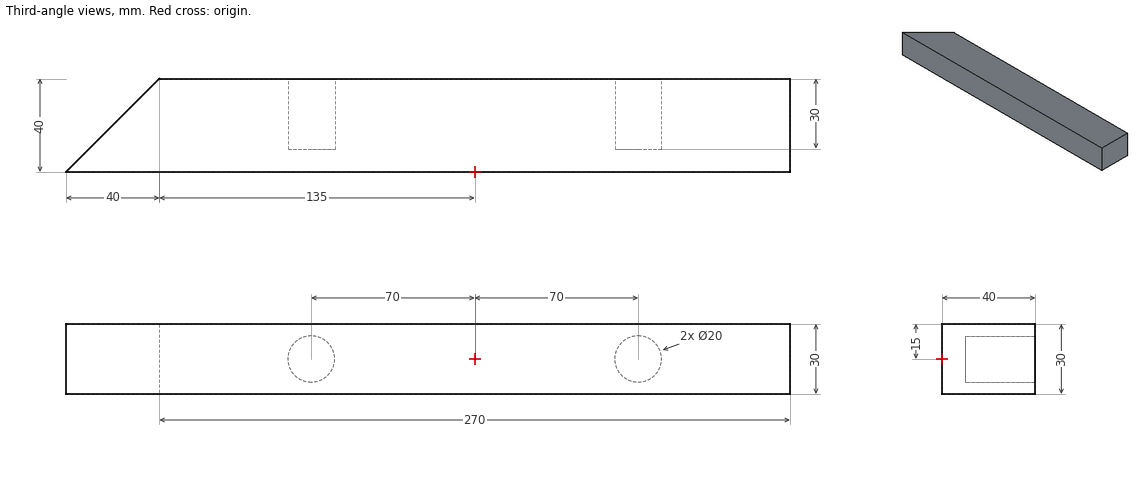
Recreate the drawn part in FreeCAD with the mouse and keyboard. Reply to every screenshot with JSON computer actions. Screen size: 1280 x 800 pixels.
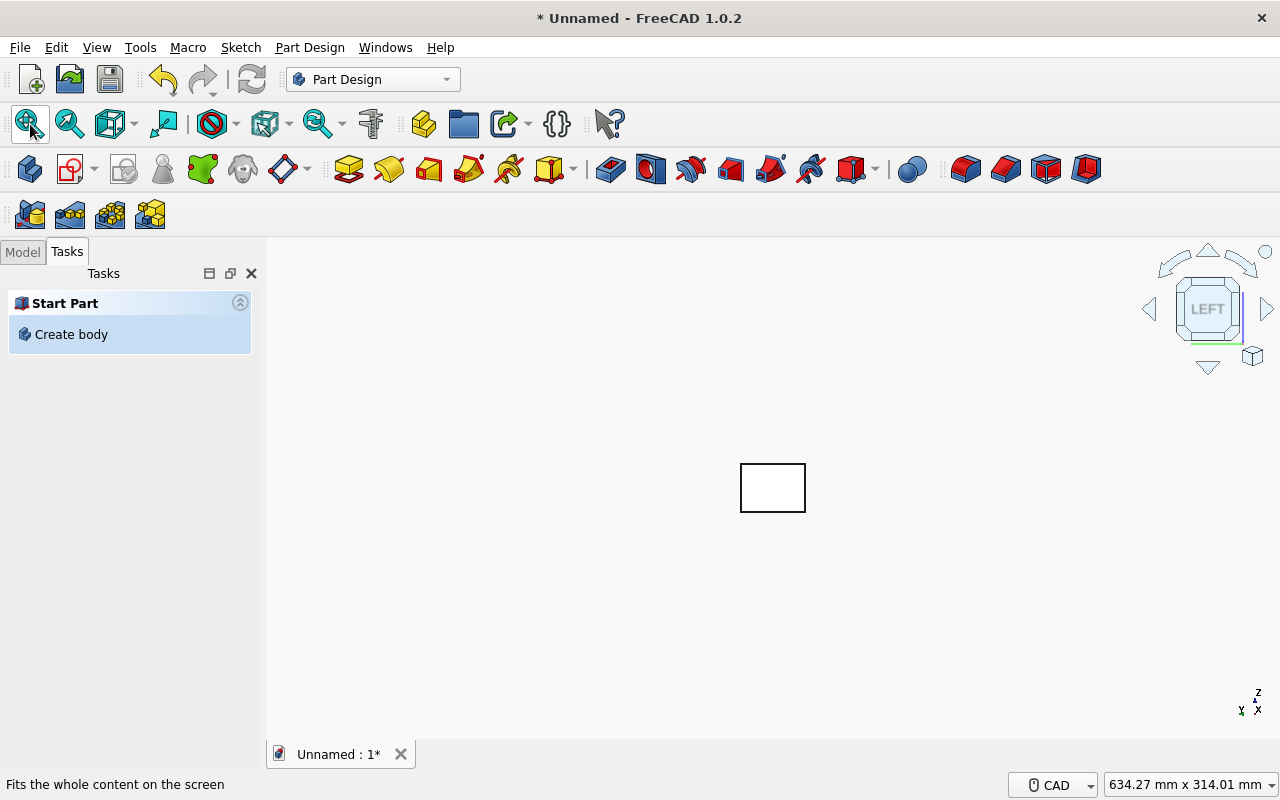
{"action": "key", "text": "0"}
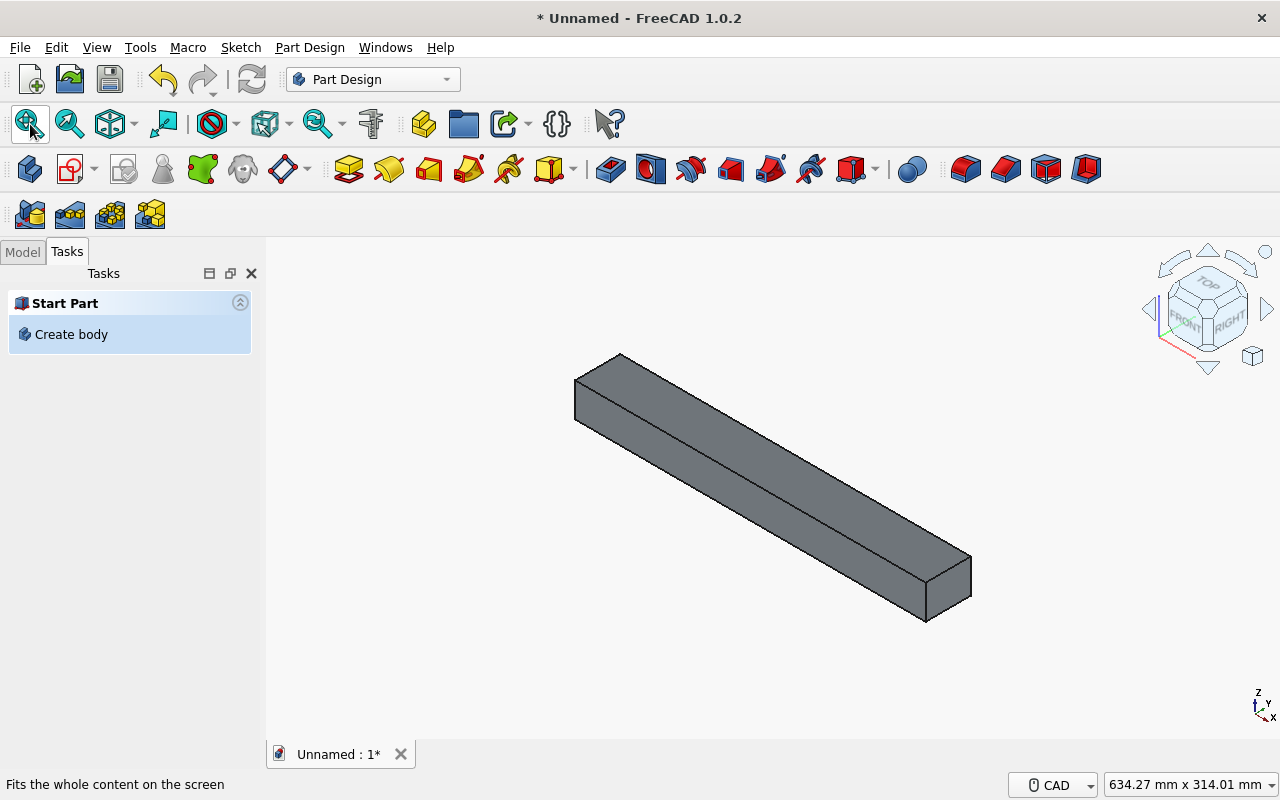
{"action": "left_click", "coordinate": [923, 554]}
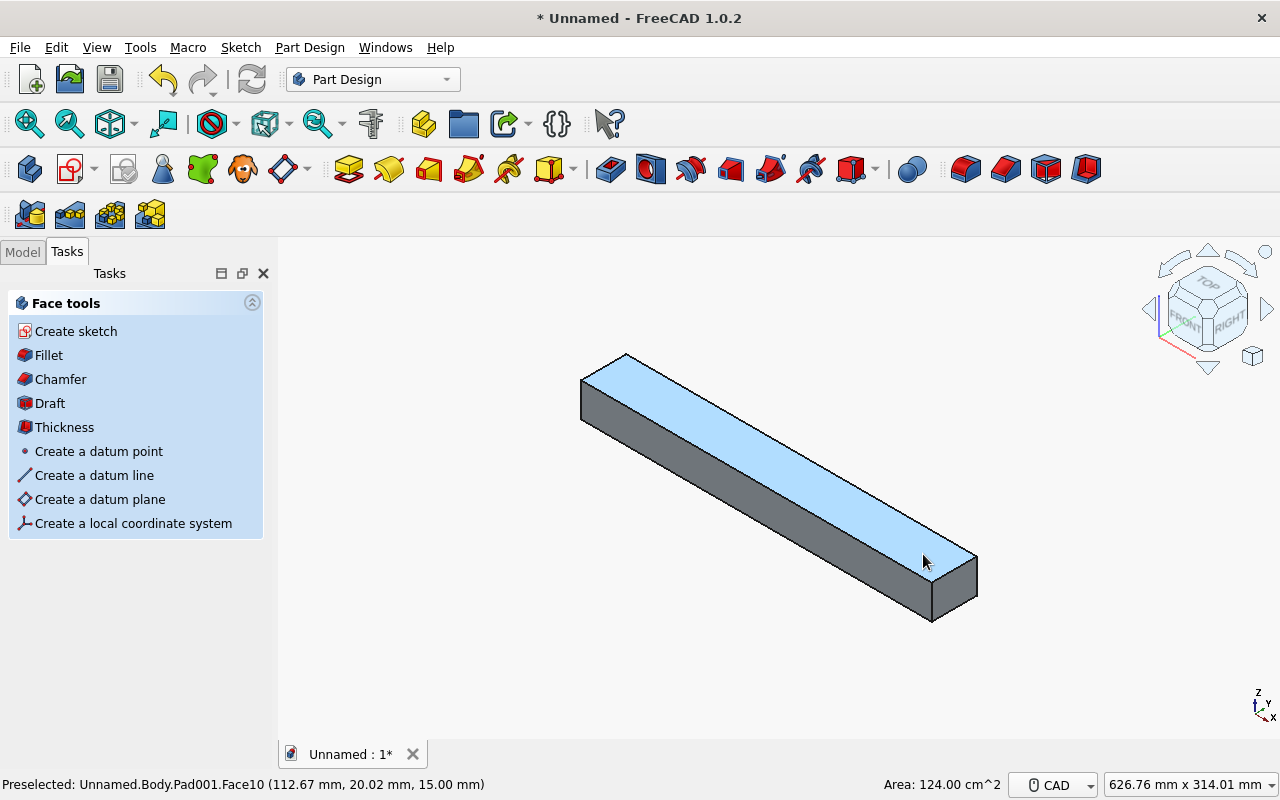
{"action": "left_click", "coordinate": [70, 170]}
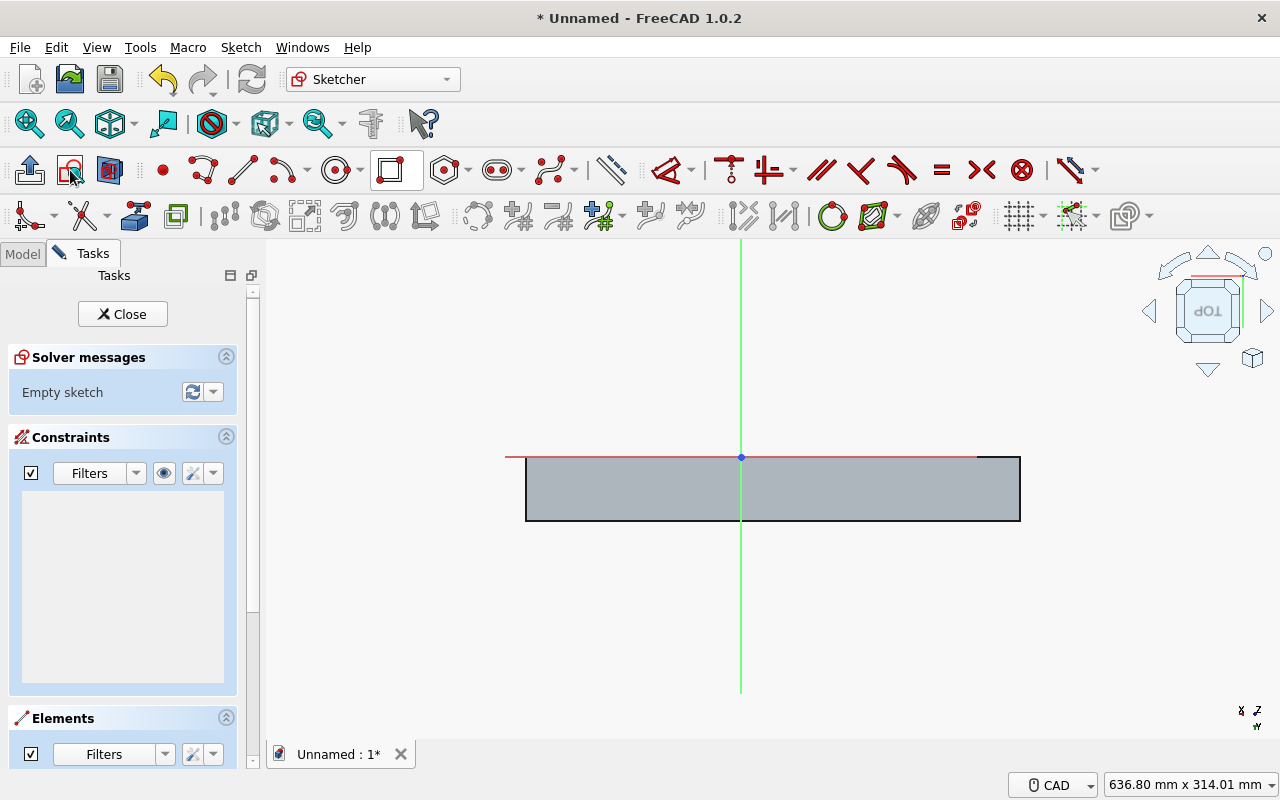
{"action": "scroll", "coordinate": [1060, 489], "scroll_direction": "up", "scroll_amount": 8}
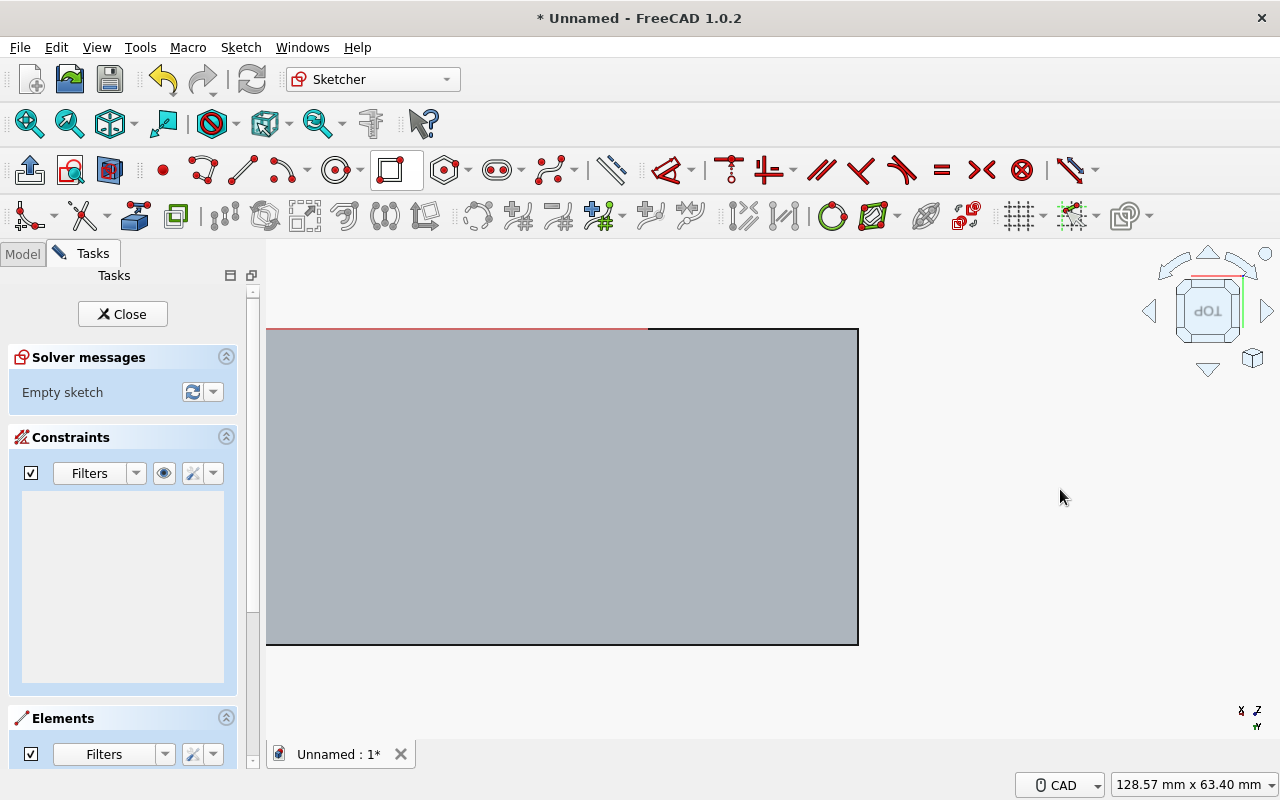
{"action": "left_click", "coordinate": [204, 170]}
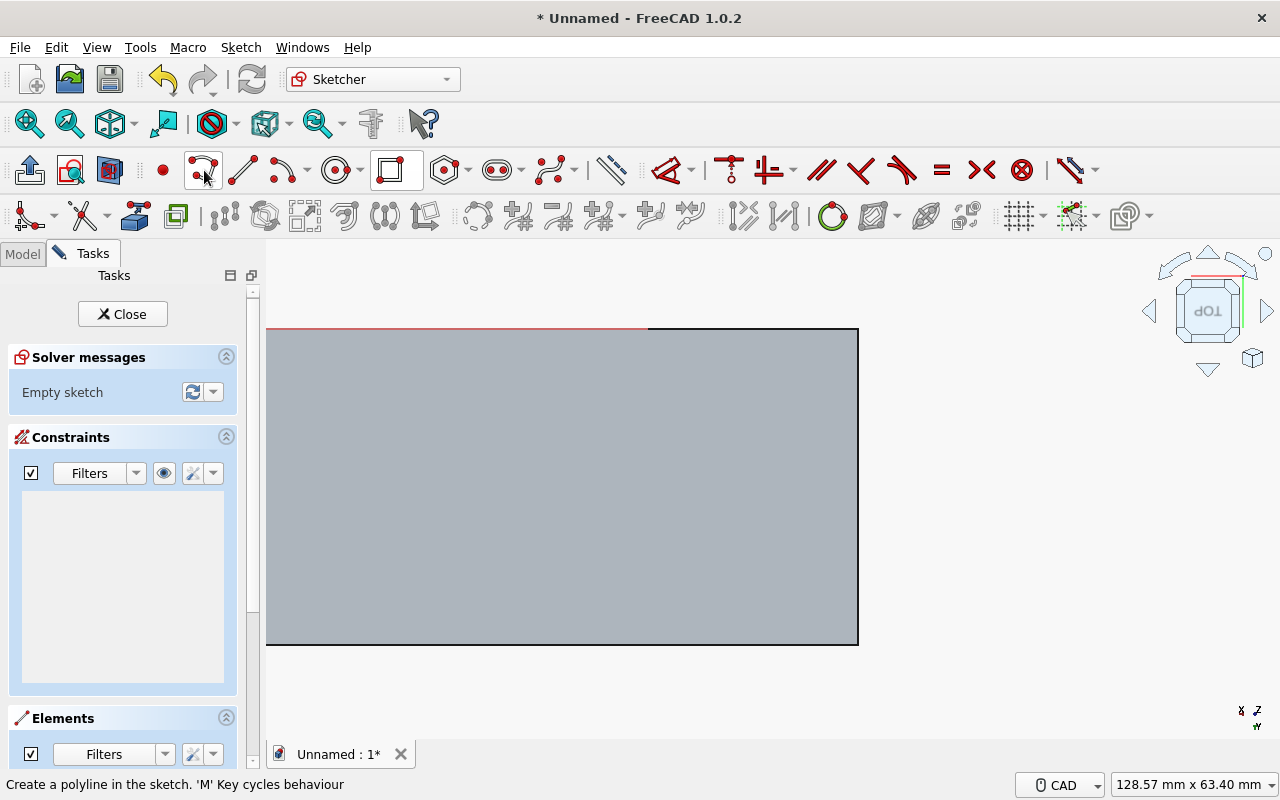
{"action": "left_click", "coordinate": [542, 645]}
{"action": "left_click", "coordinate": [858, 645]}
{"action": "left_click", "coordinate": [858, 329]}
{"action": "left_click", "coordinate": [542, 646]}
{"action": "key", "text": "Escape"}
{"action": "key", "text": "Escape"}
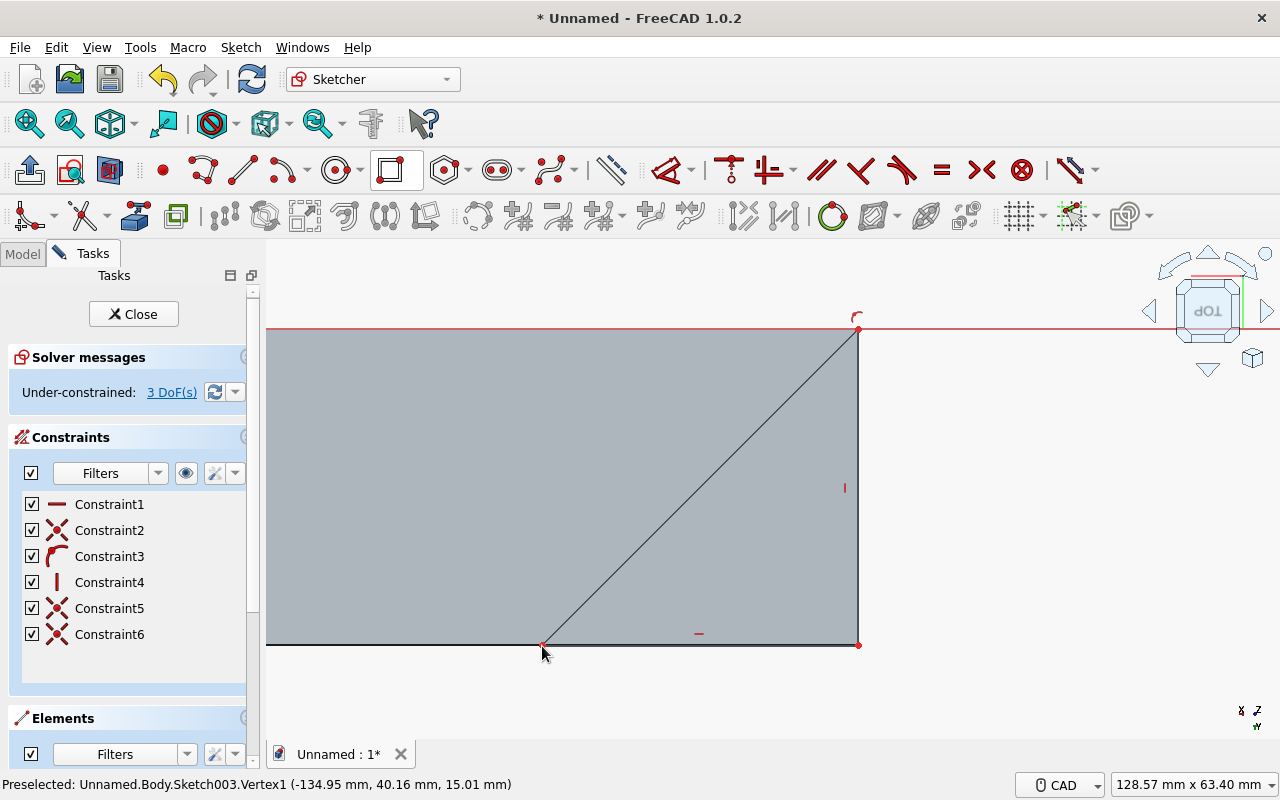
{"action": "left_click", "coordinate": [666, 170]}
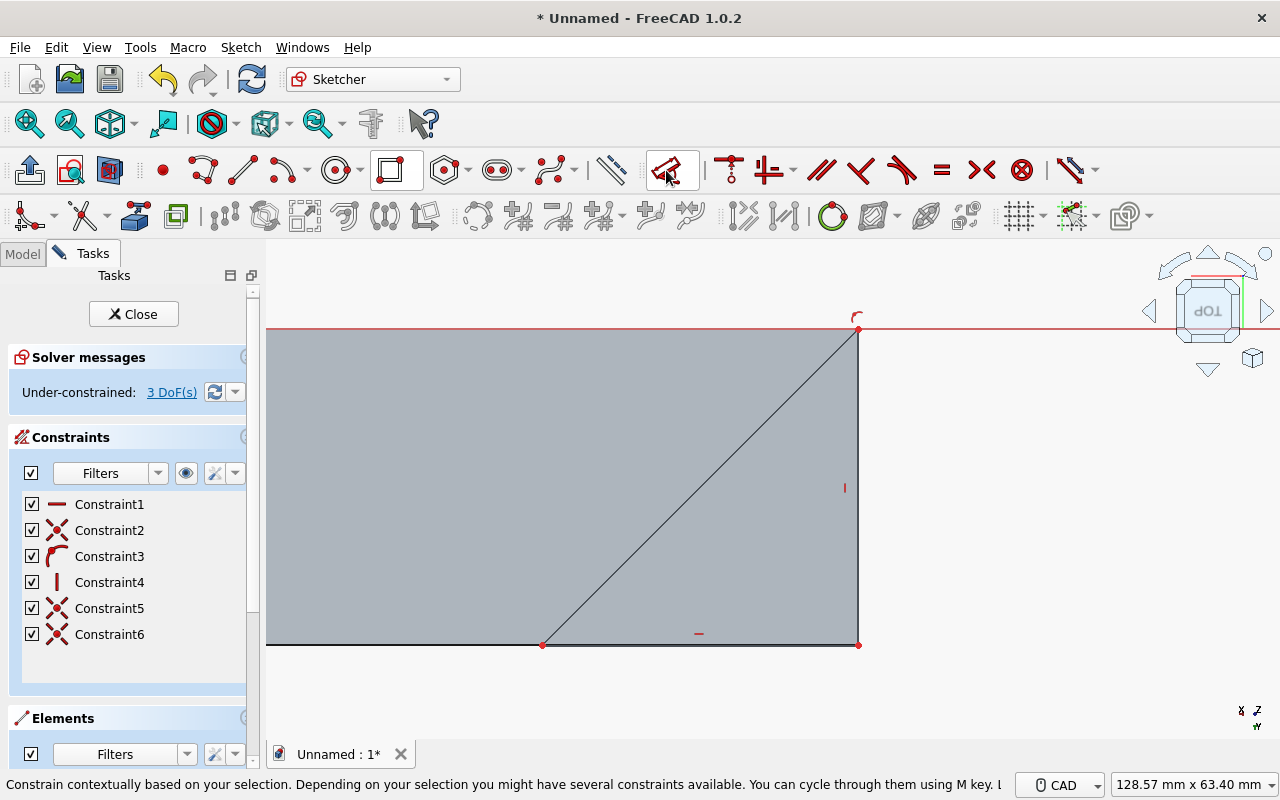
{"action": "left_click", "coordinate": [637, 646]}
{"action": "left_click", "coordinate": [700, 680]}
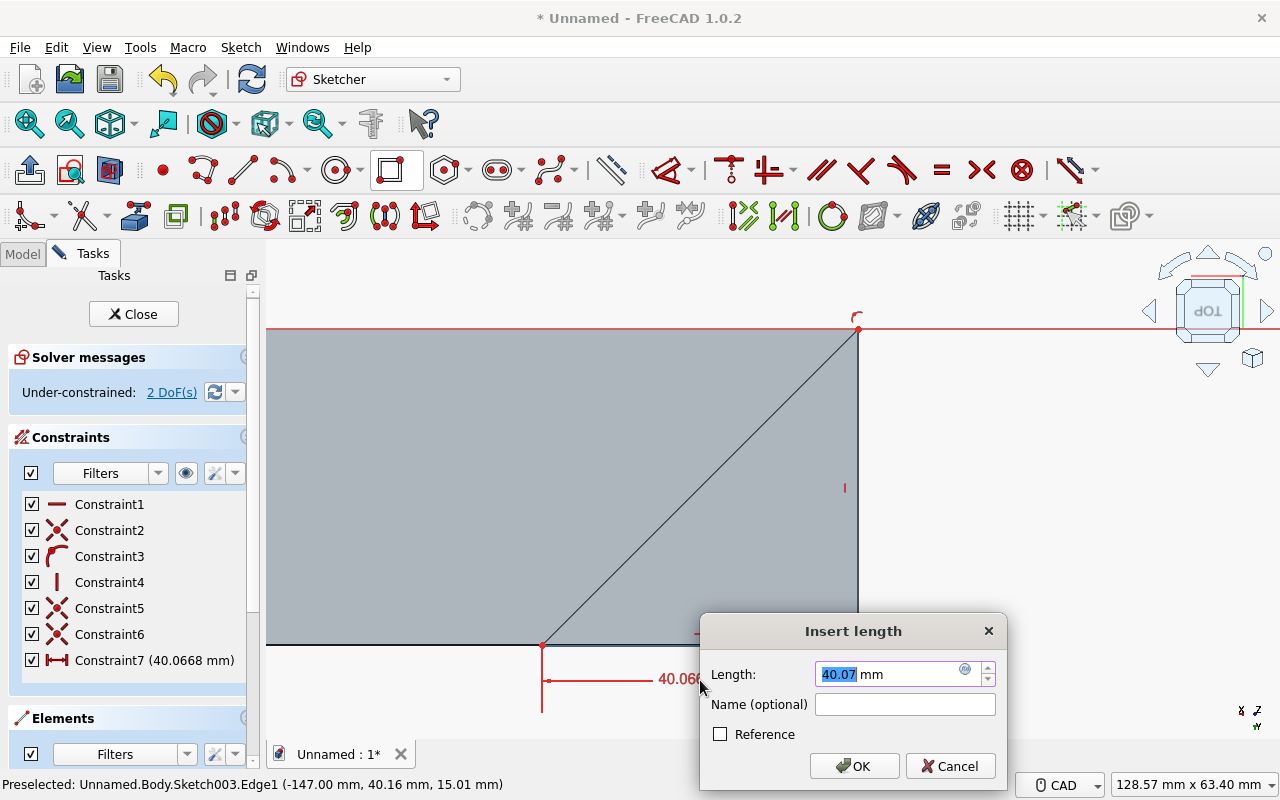
{"action": "type", "text": "40"}
{"action": "key", "text": "Return"}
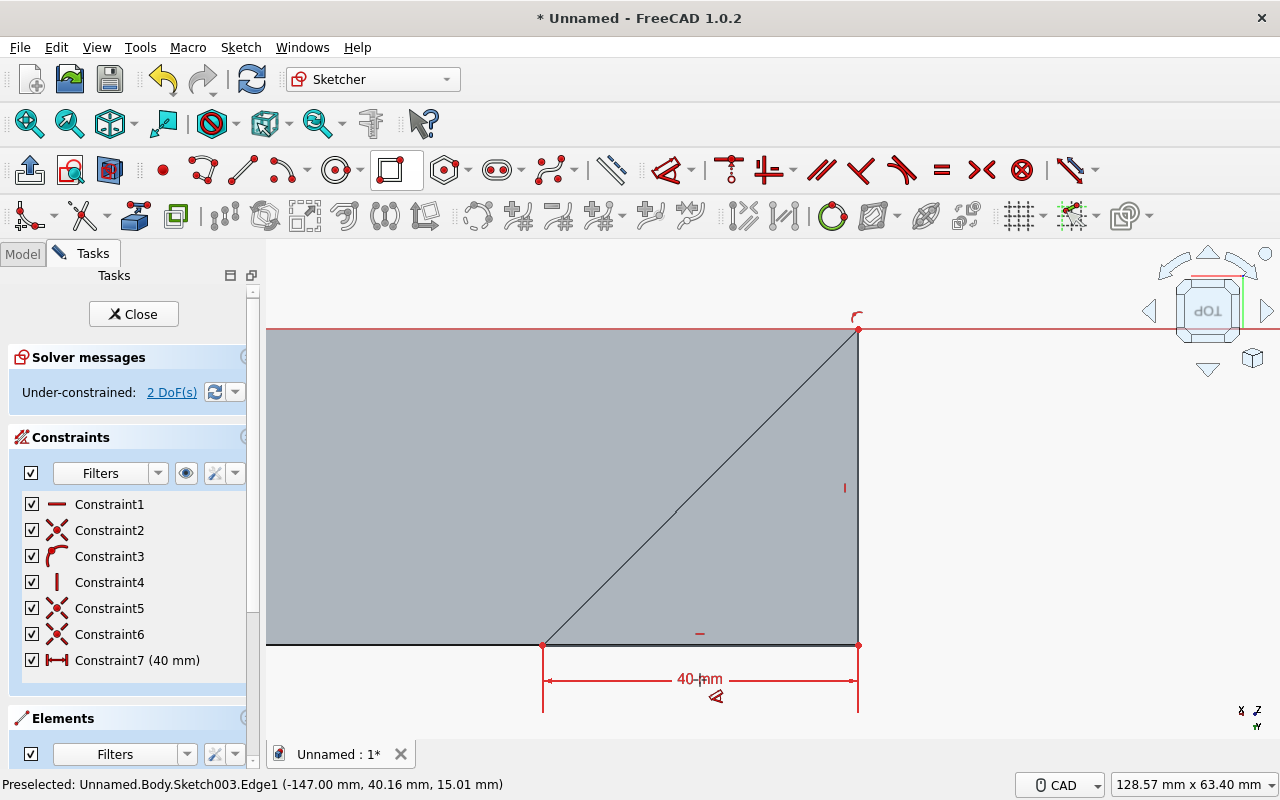
{"action": "left_click", "coordinate": [858, 551]}
{"action": "left_click", "coordinate": [892, 488]}